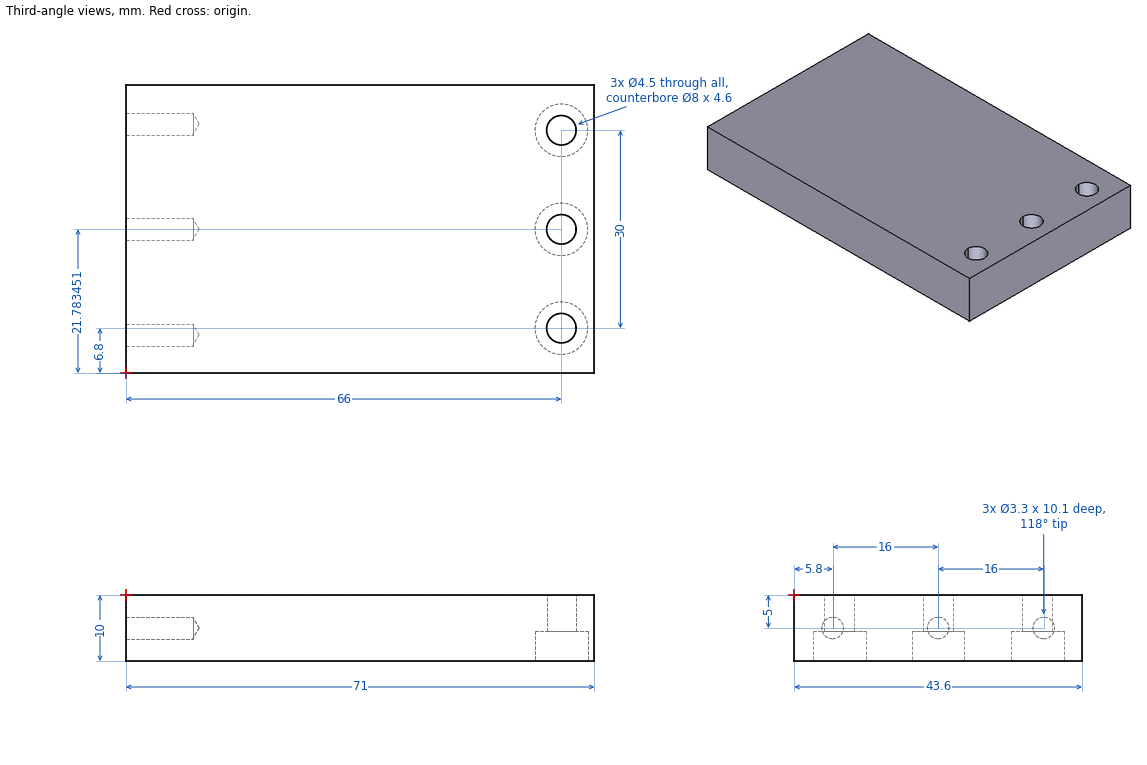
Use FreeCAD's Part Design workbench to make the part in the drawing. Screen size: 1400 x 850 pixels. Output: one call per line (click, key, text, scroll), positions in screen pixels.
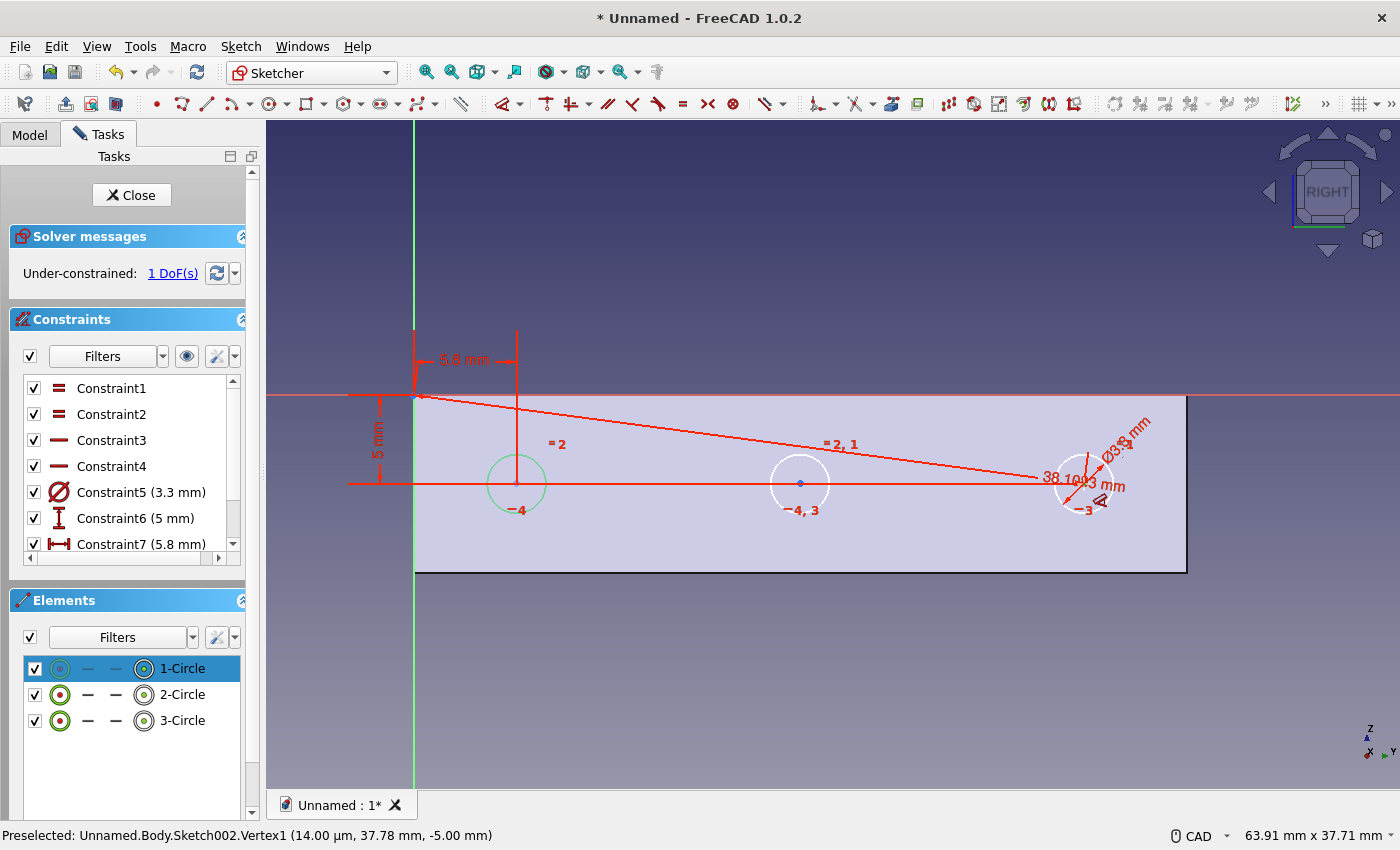
click(800, 484)
click(942, 518)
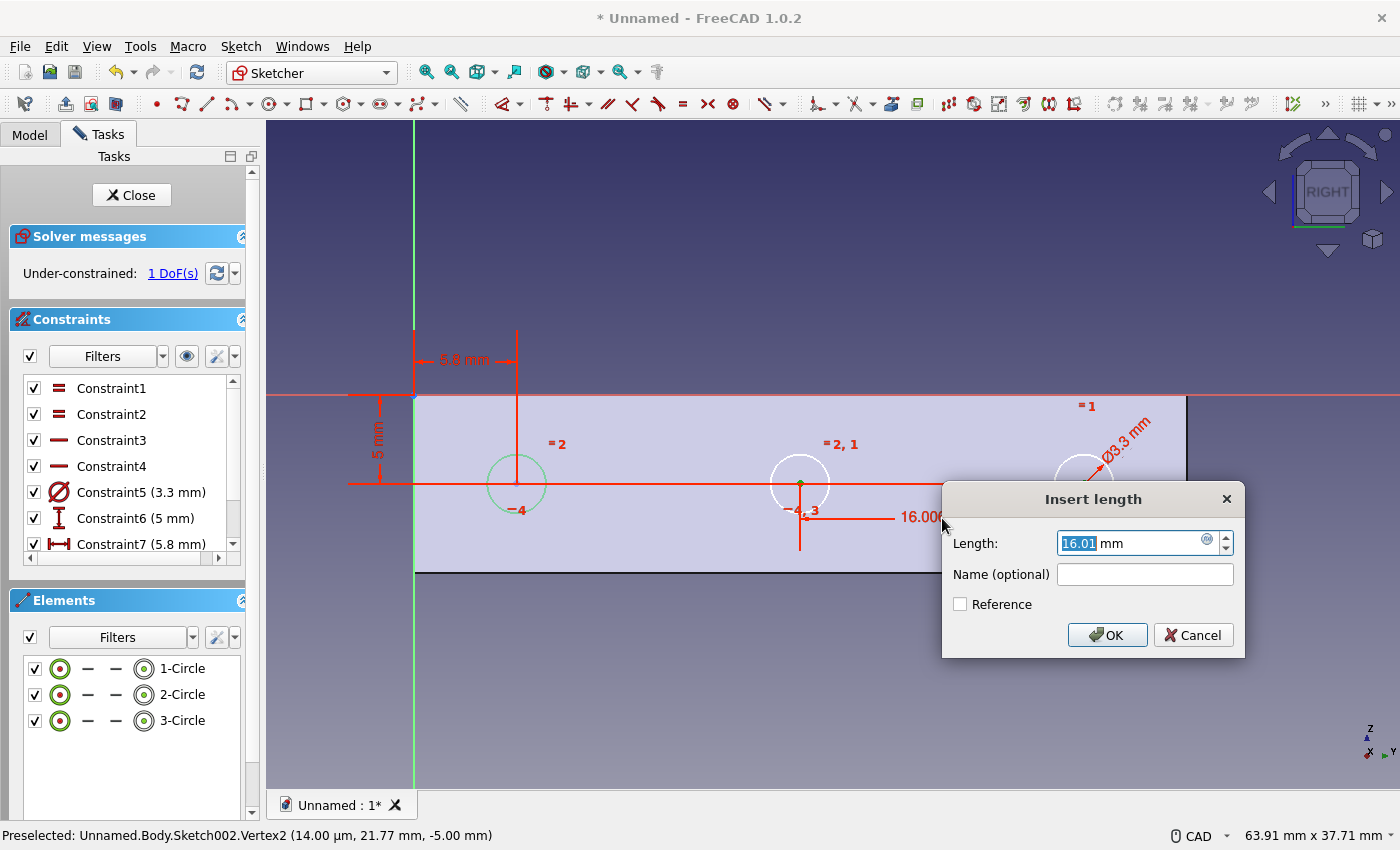
text(16)
key(Return)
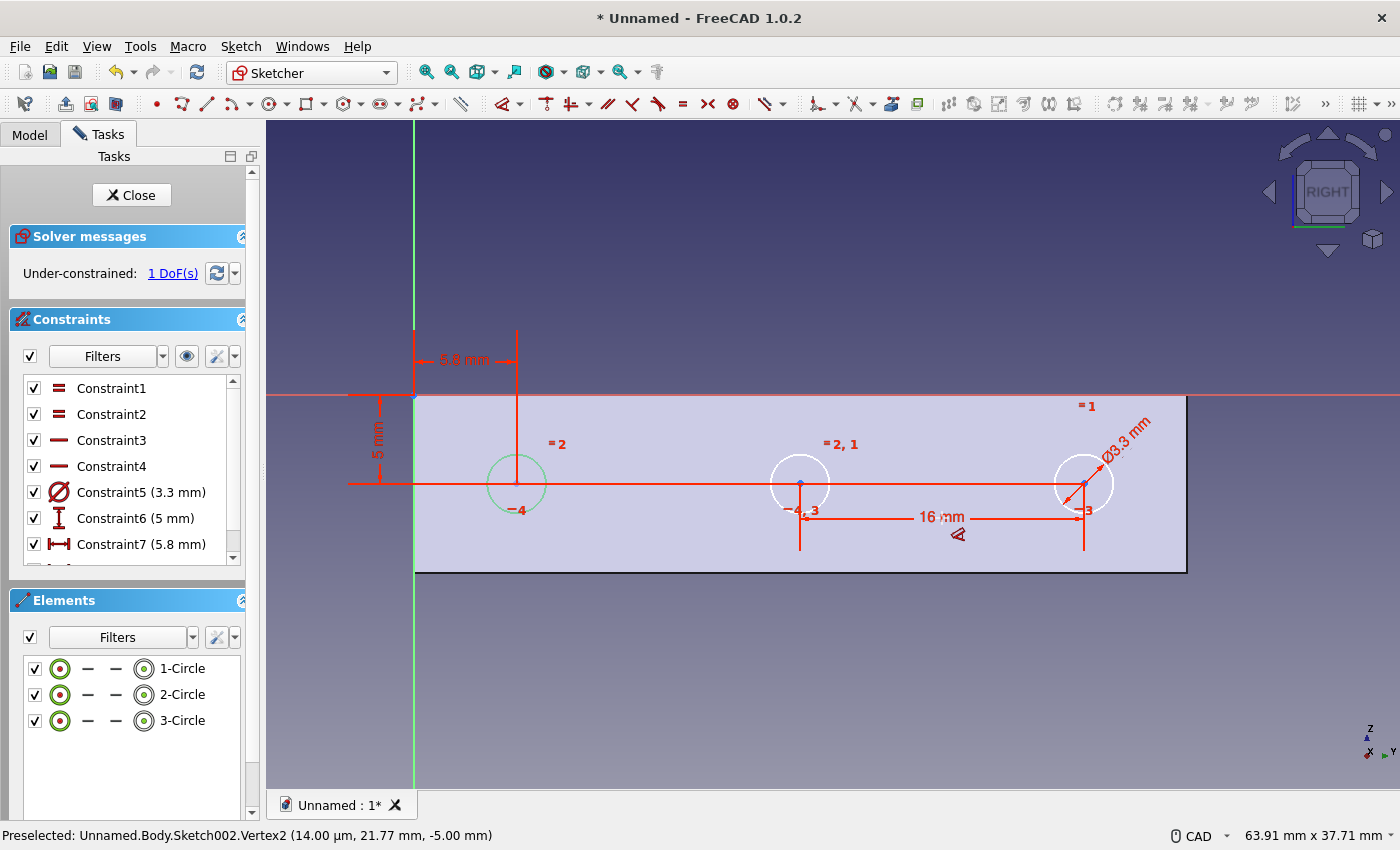
click(800, 484)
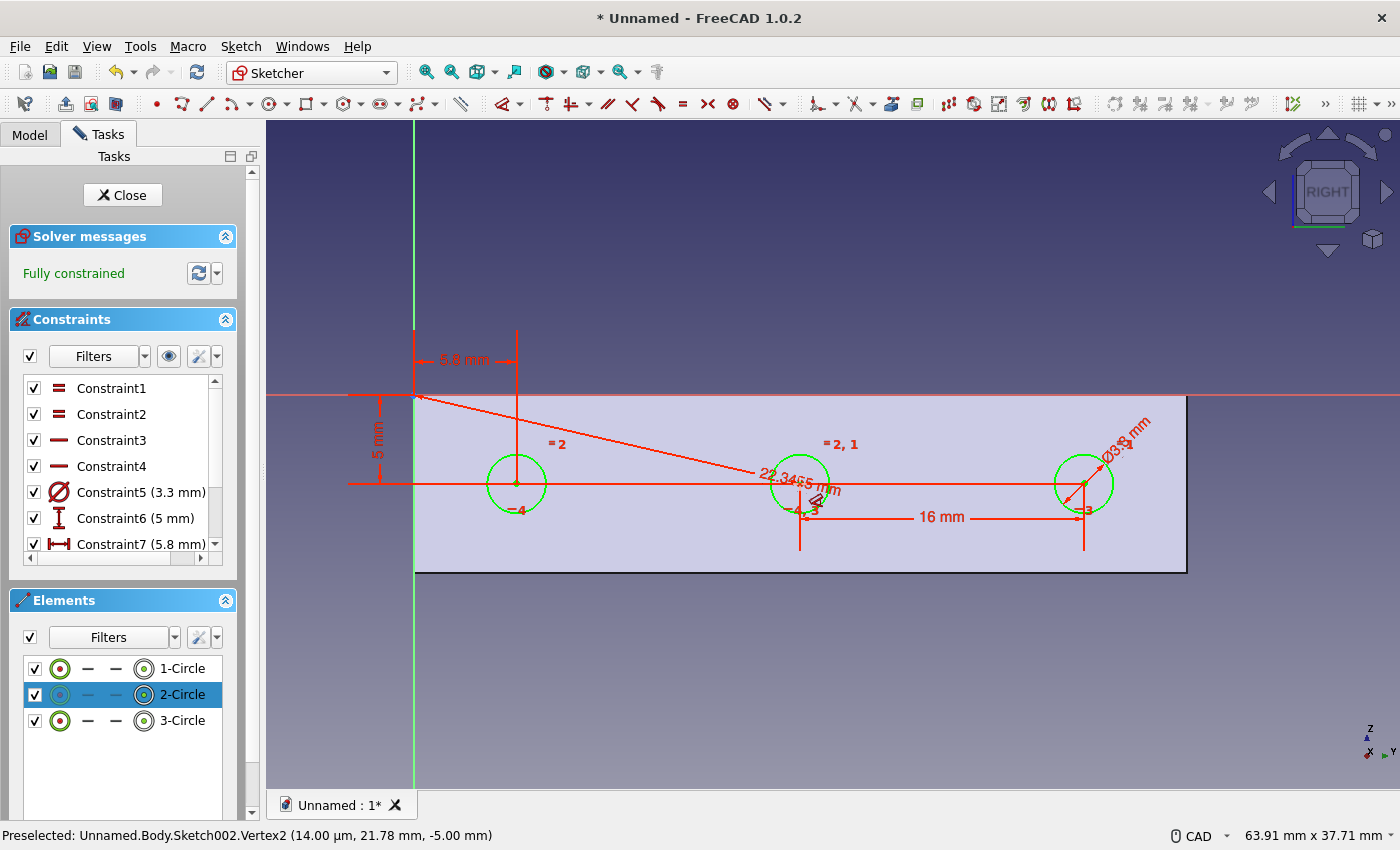
click(517, 484)
click(658, 518)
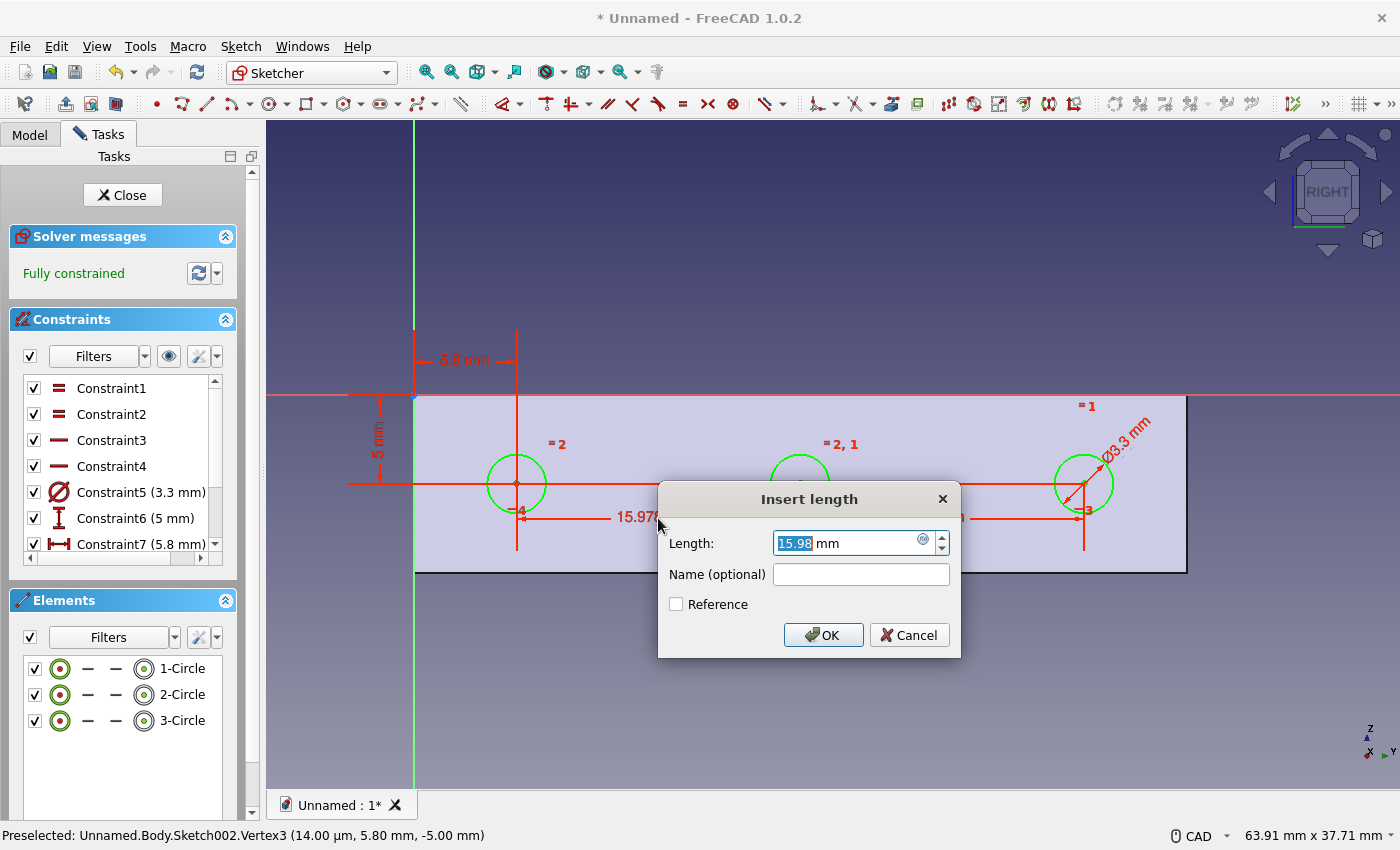
text(16)
key(Return)
key(Escape)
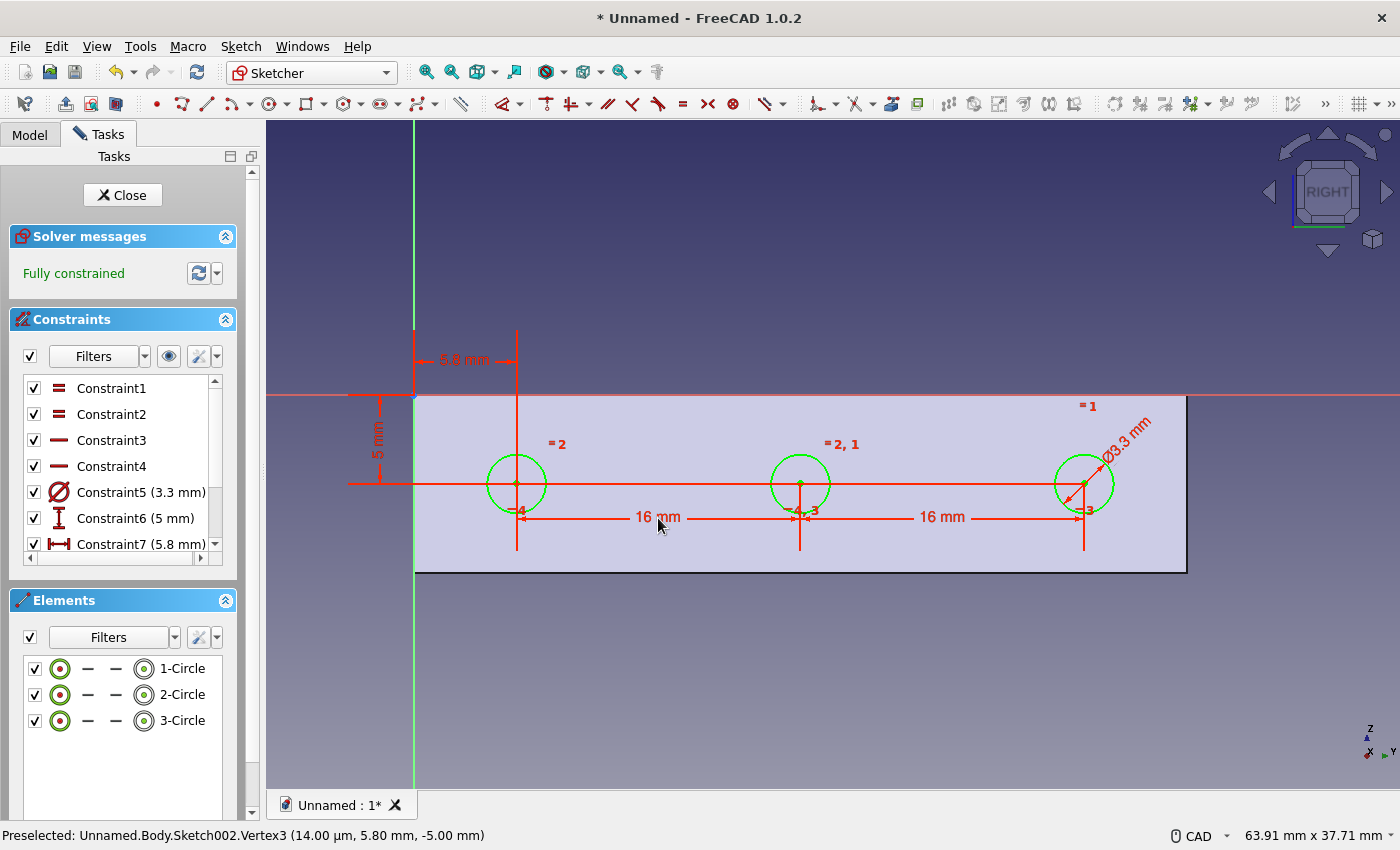
click(123, 195)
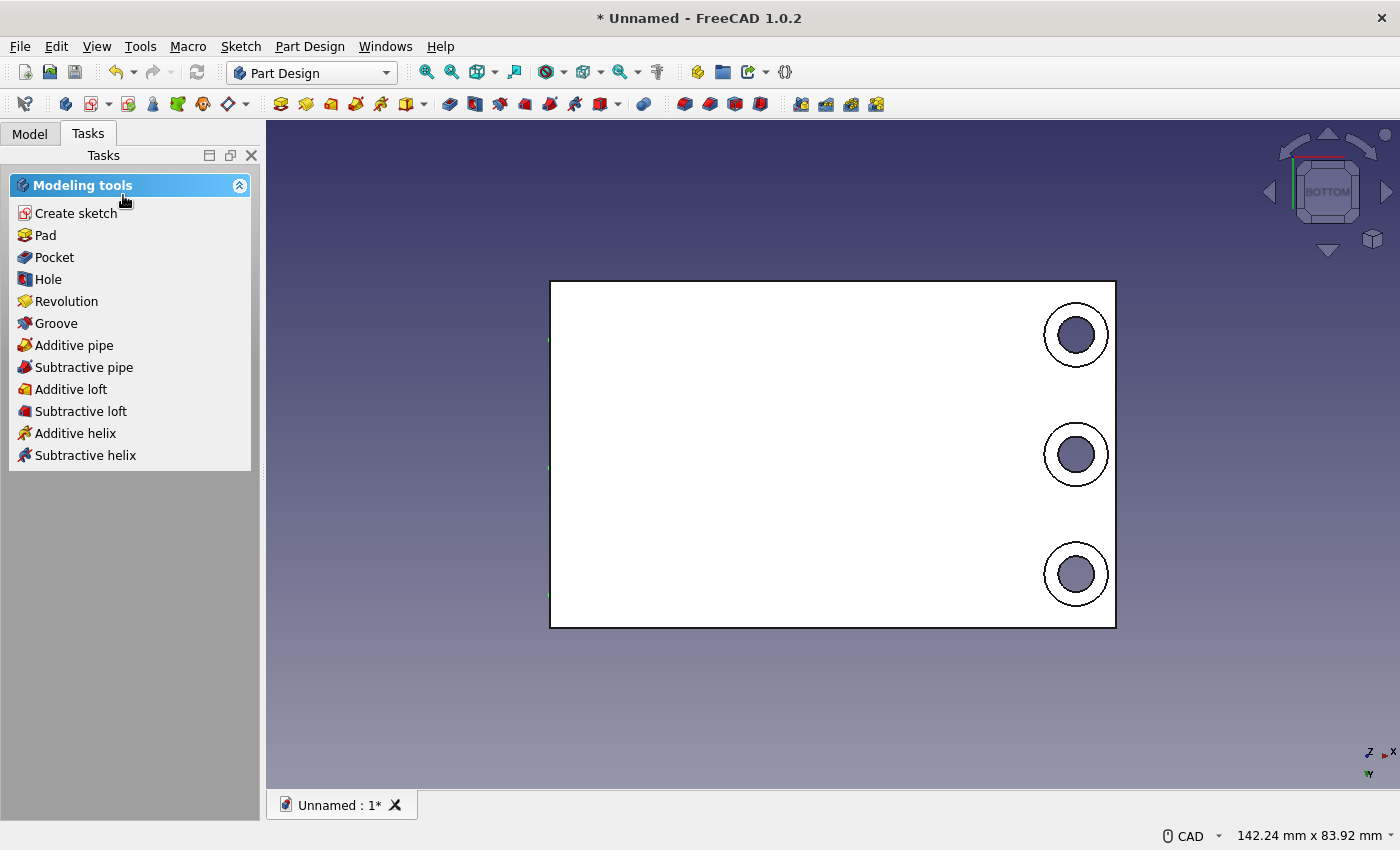
click(475, 104)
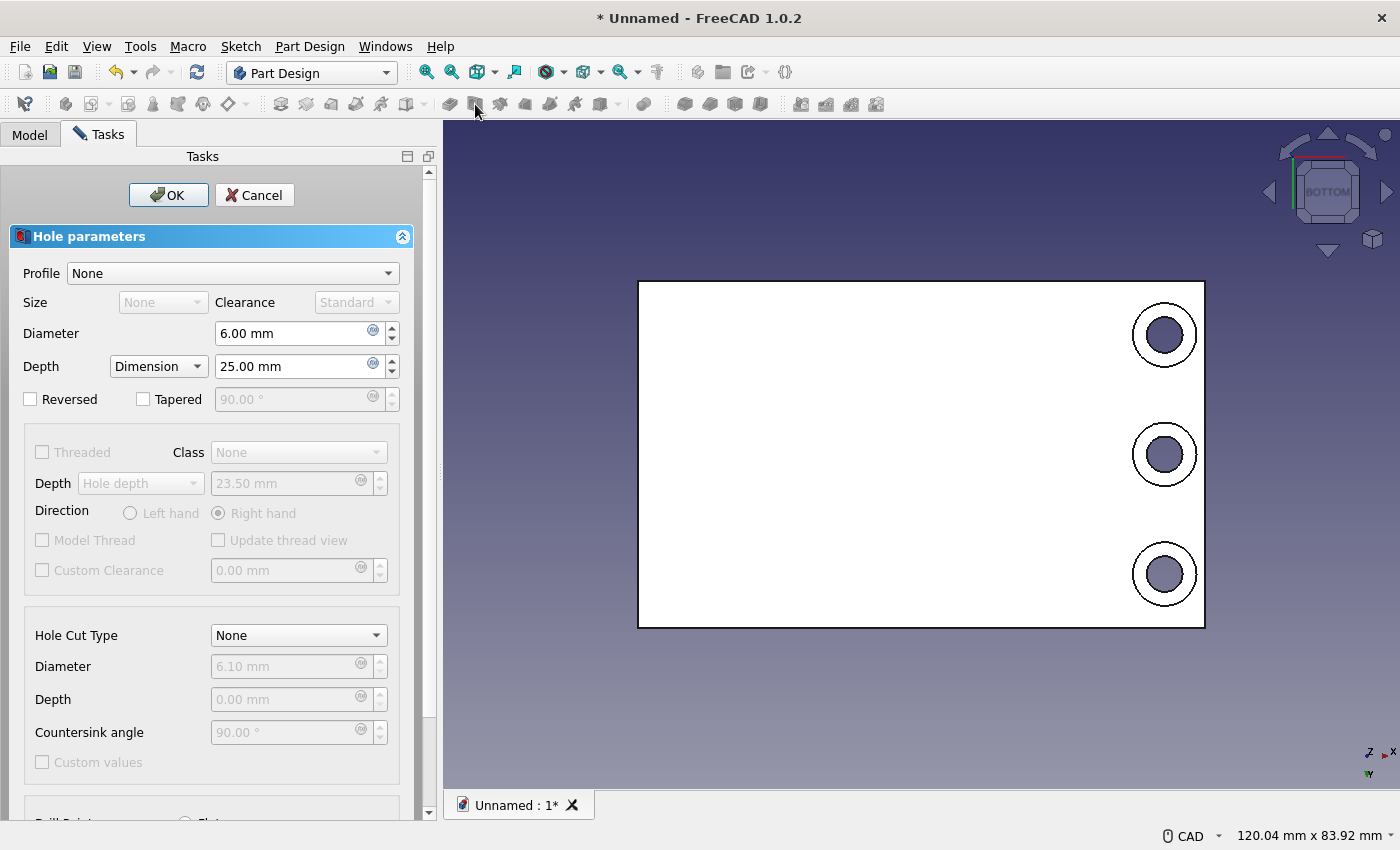
triple_click(300, 334)